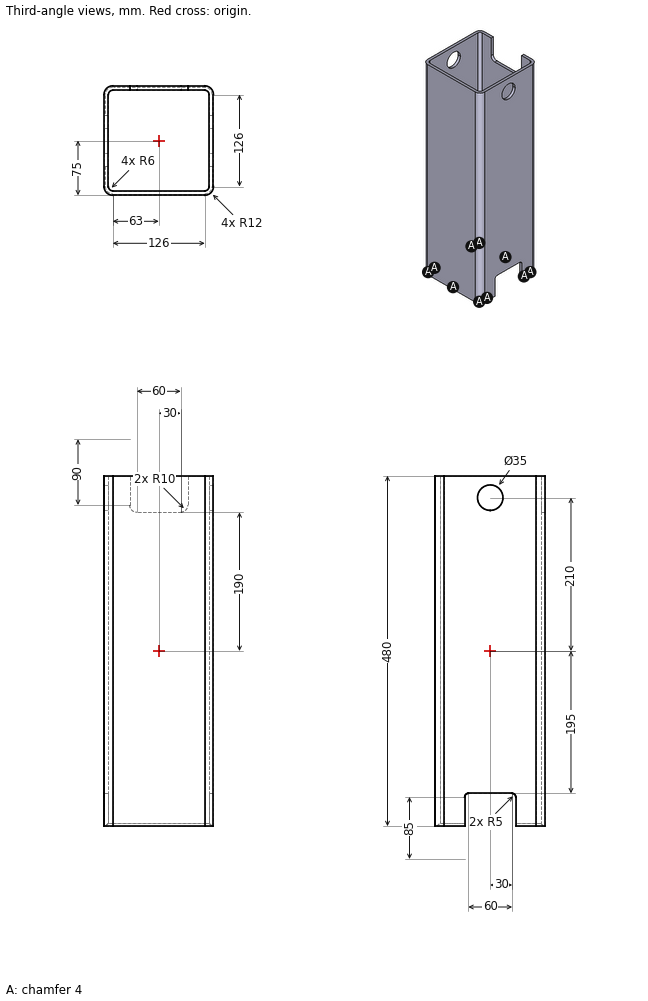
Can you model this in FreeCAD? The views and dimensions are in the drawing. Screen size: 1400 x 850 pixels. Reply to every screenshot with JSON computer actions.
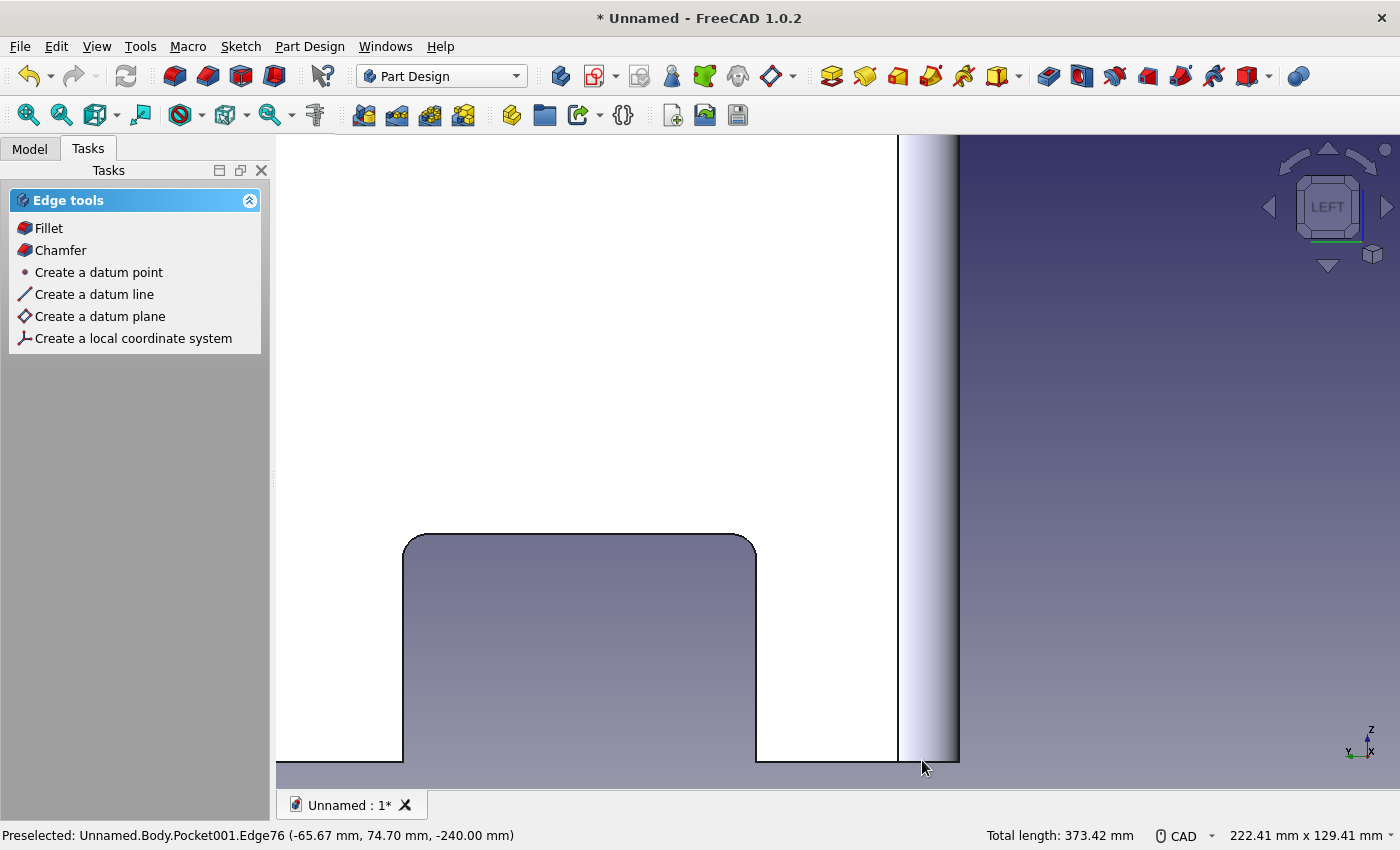
{"action": "key", "text": "v f"}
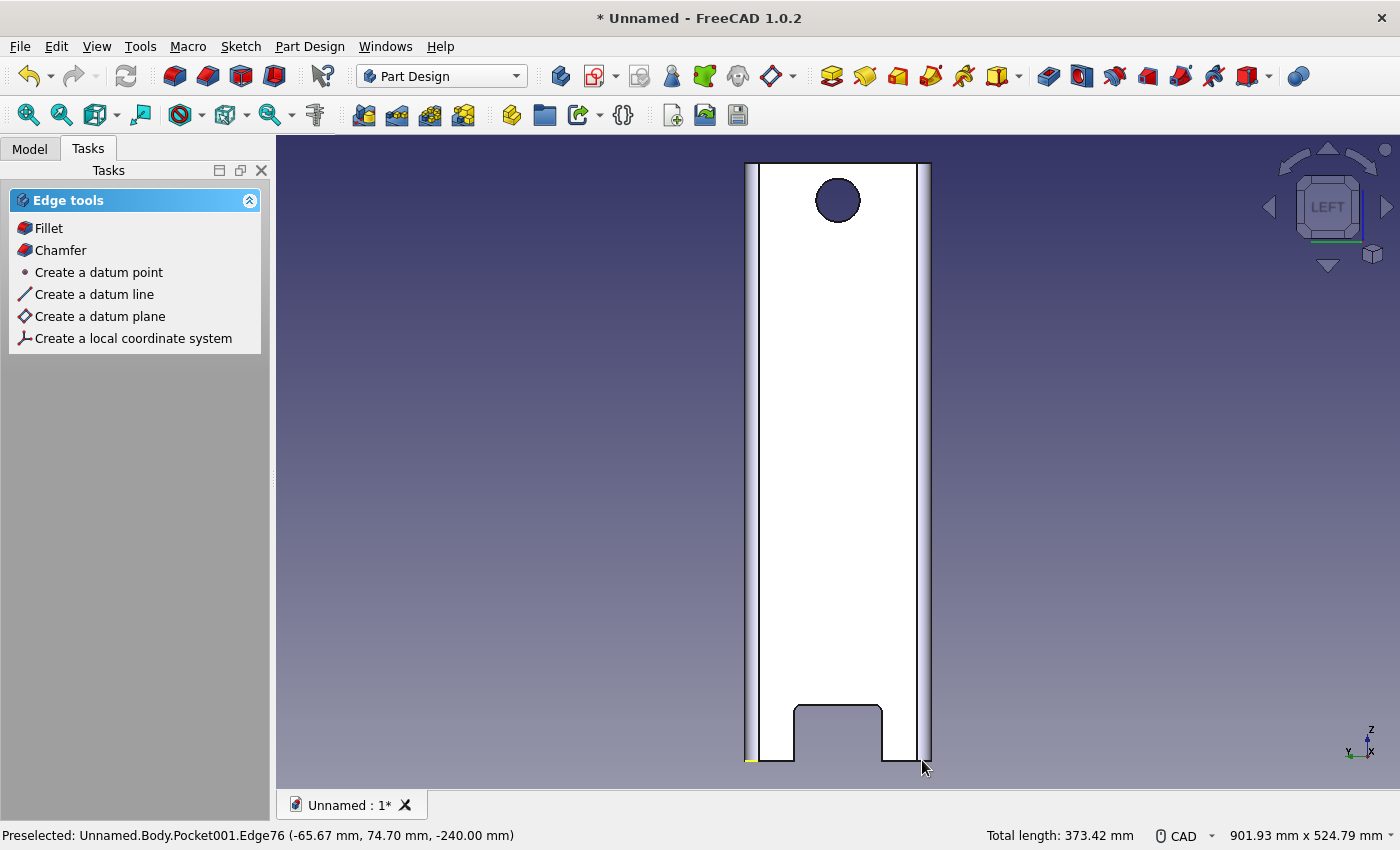
{"action": "key", "text": "v 3"}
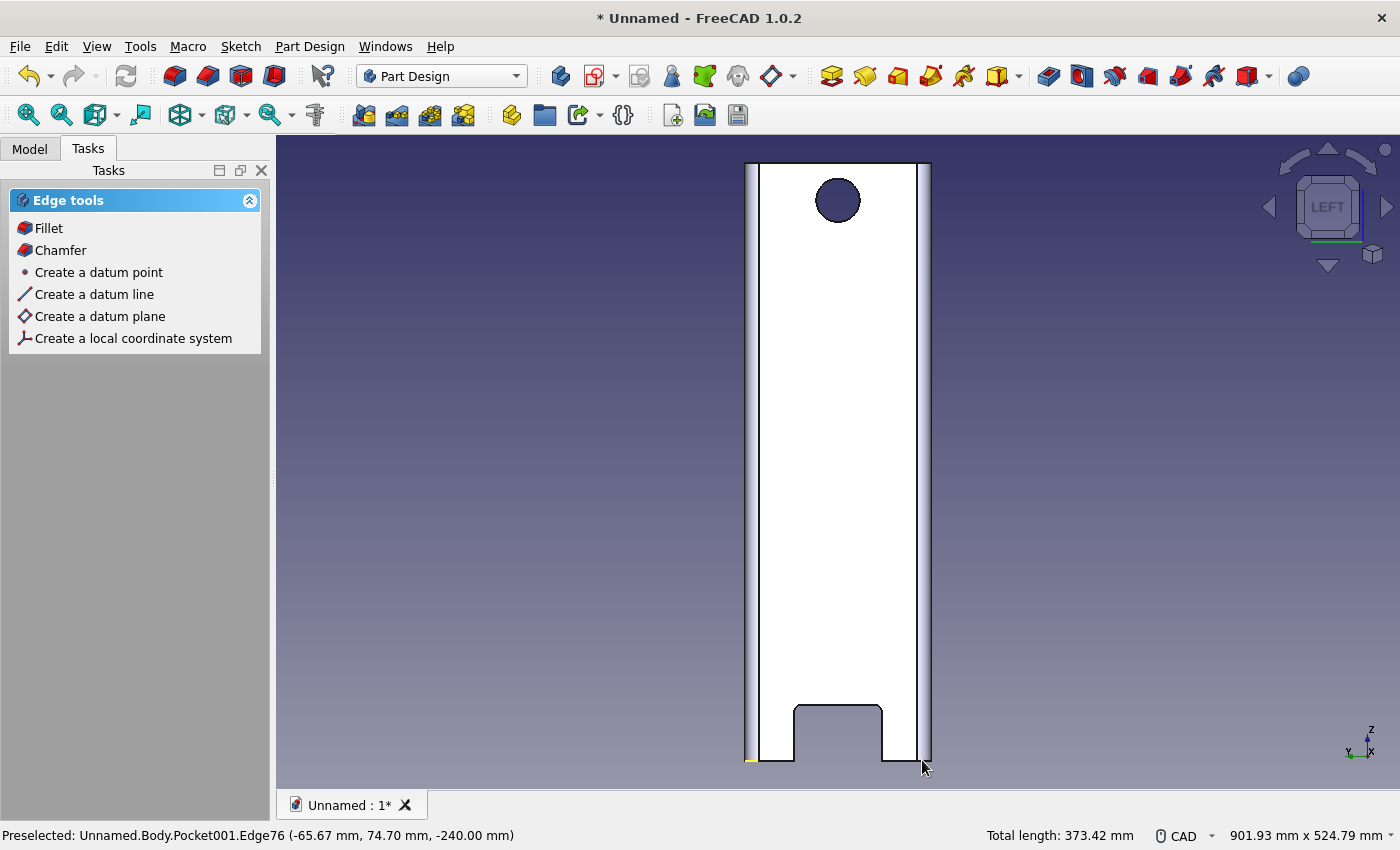
{"action": "key", "text": "0"}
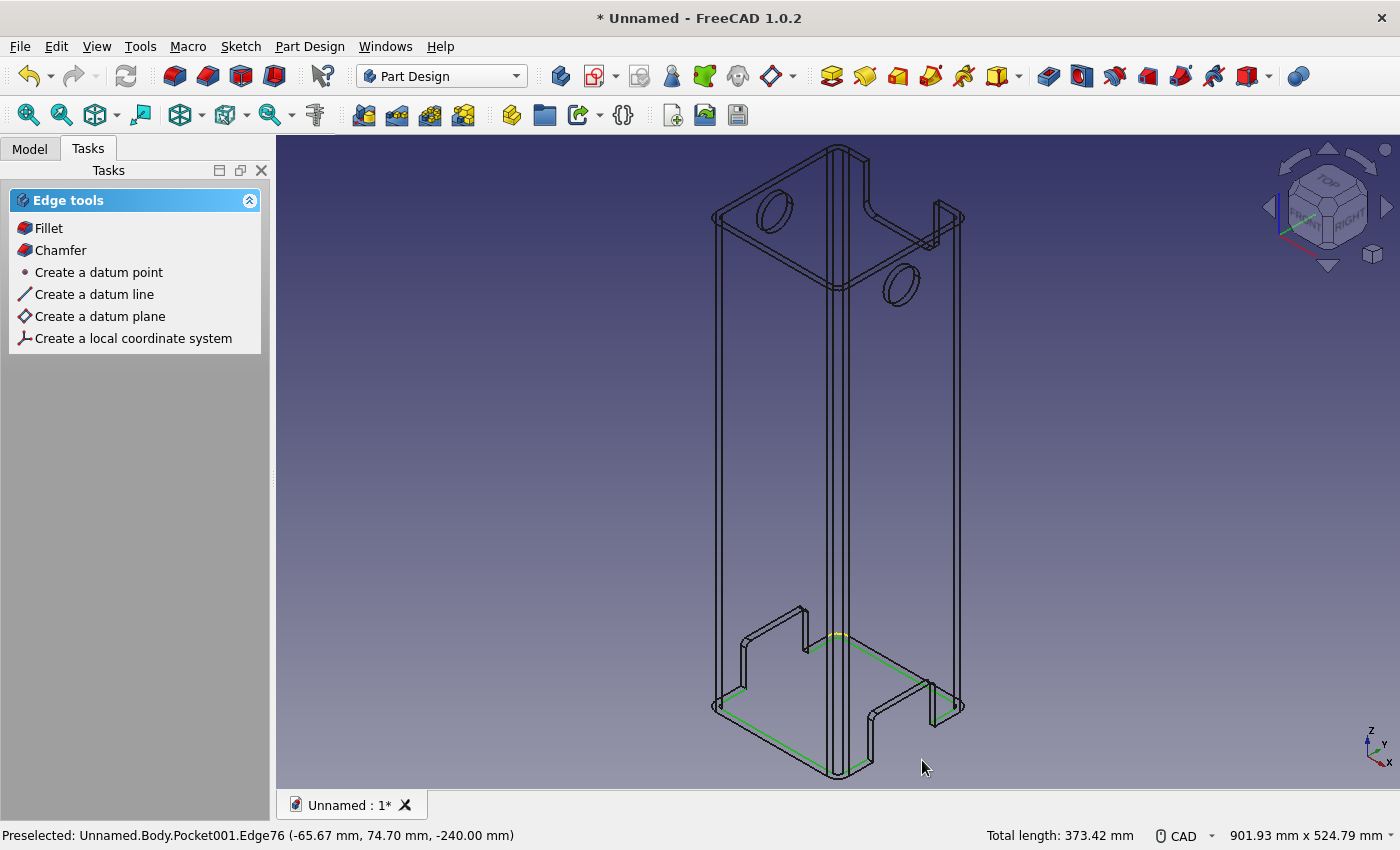
{"action": "scroll", "coordinate": [719, 705], "scroll_direction": "up", "scroll_amount": 7}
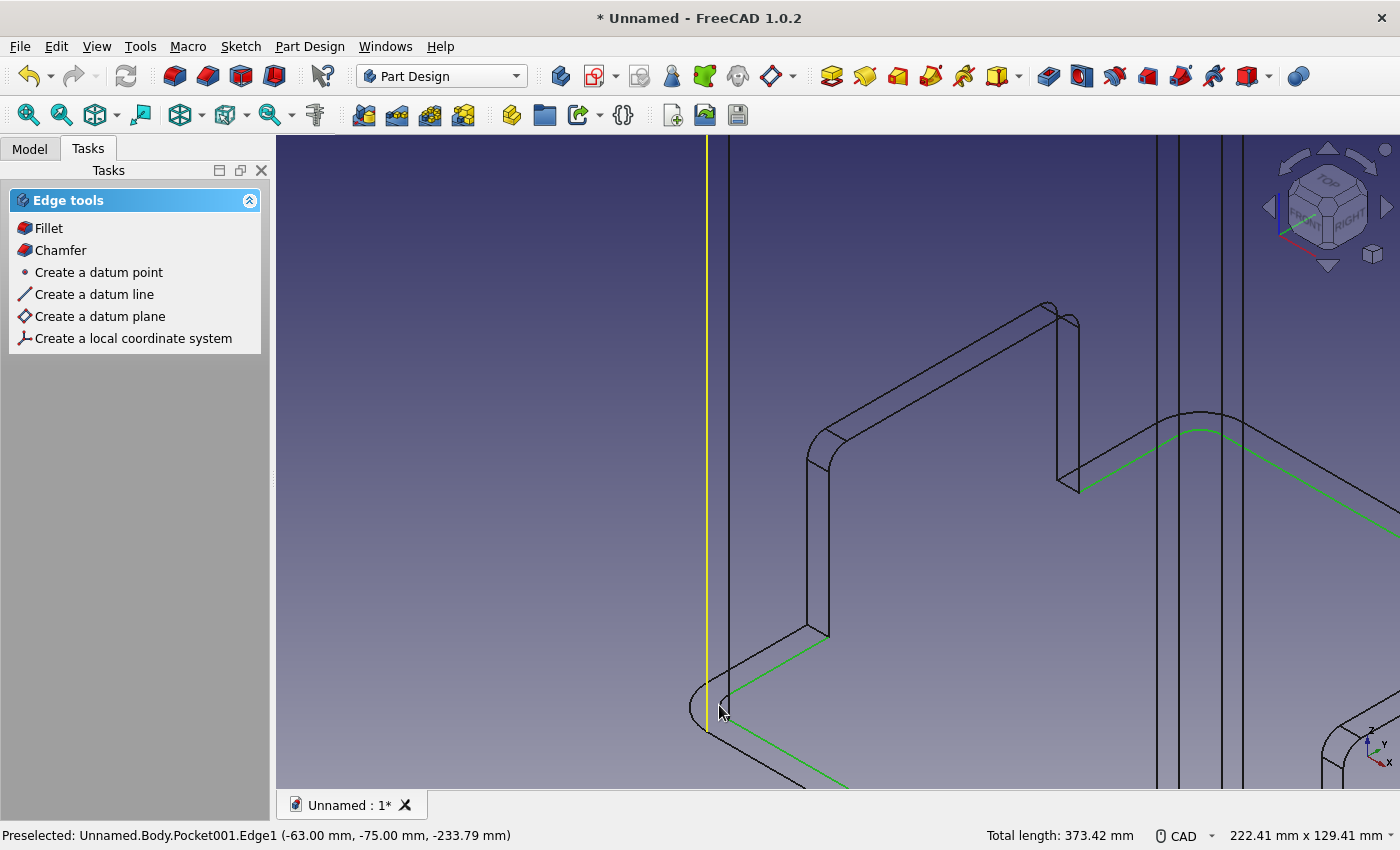
{"action": "left_click", "coordinate": [720, 706], "text": "ctrl"}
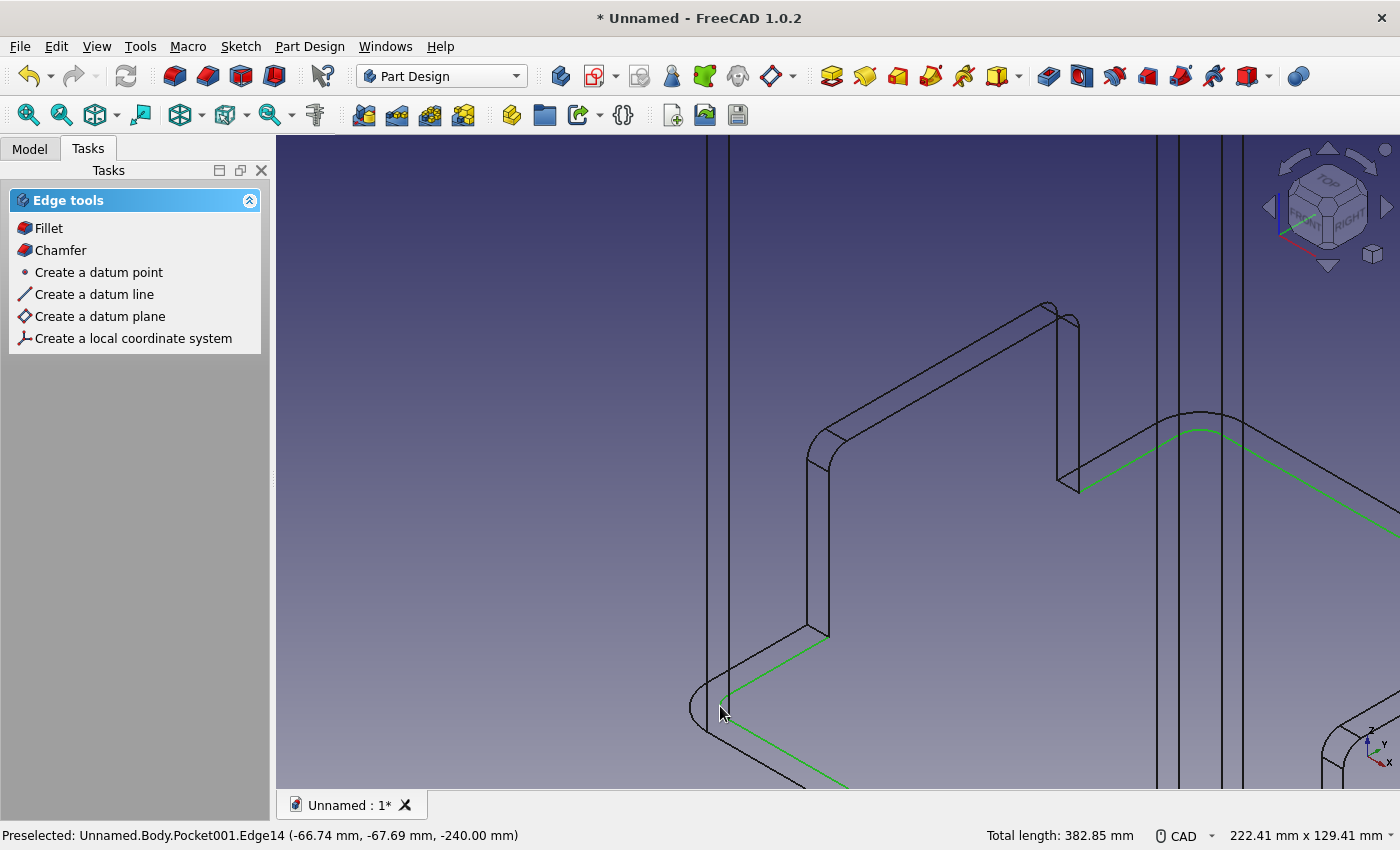
{"action": "left_click", "coordinate": [29, 116]}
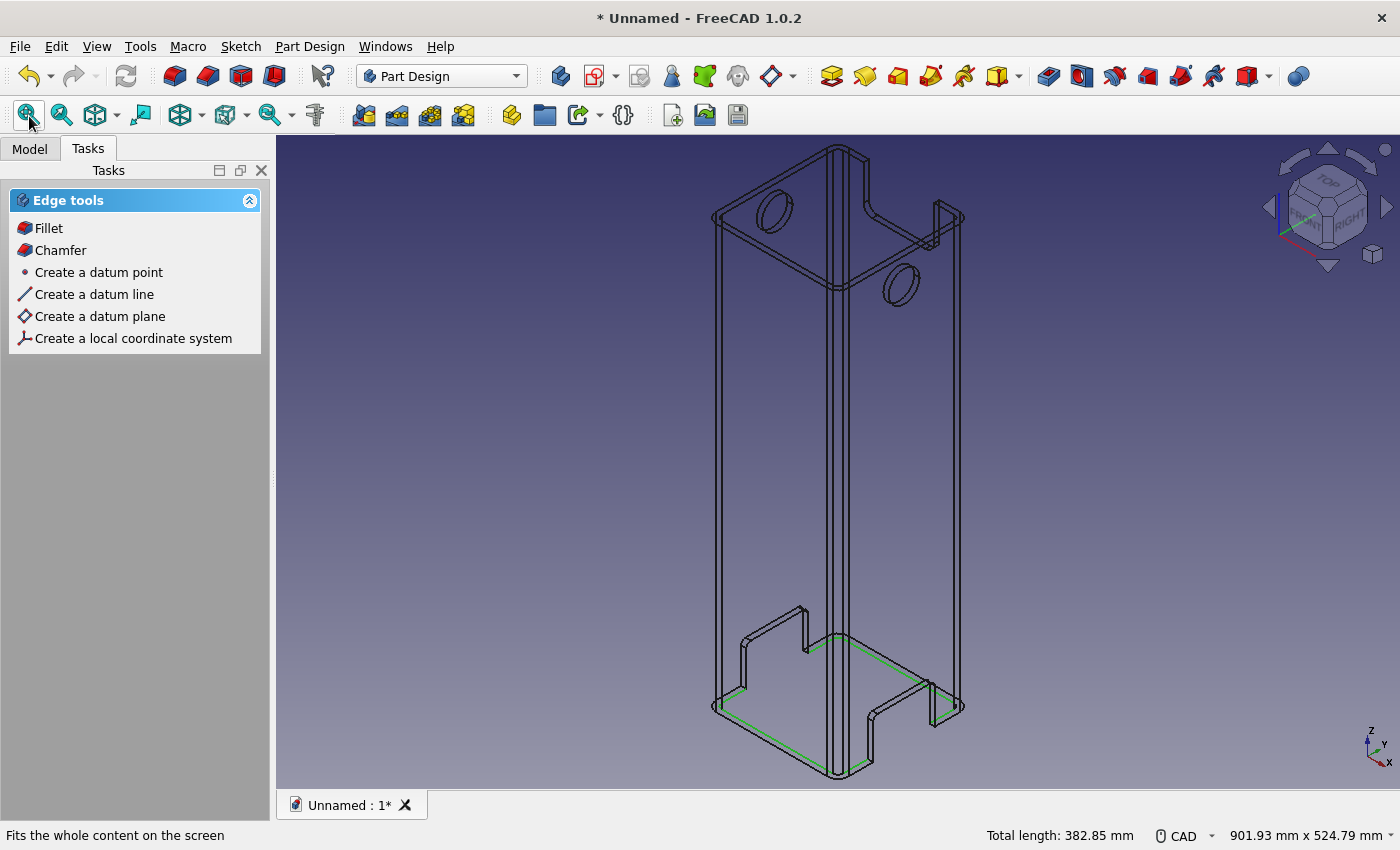
{"action": "key", "text": "2"}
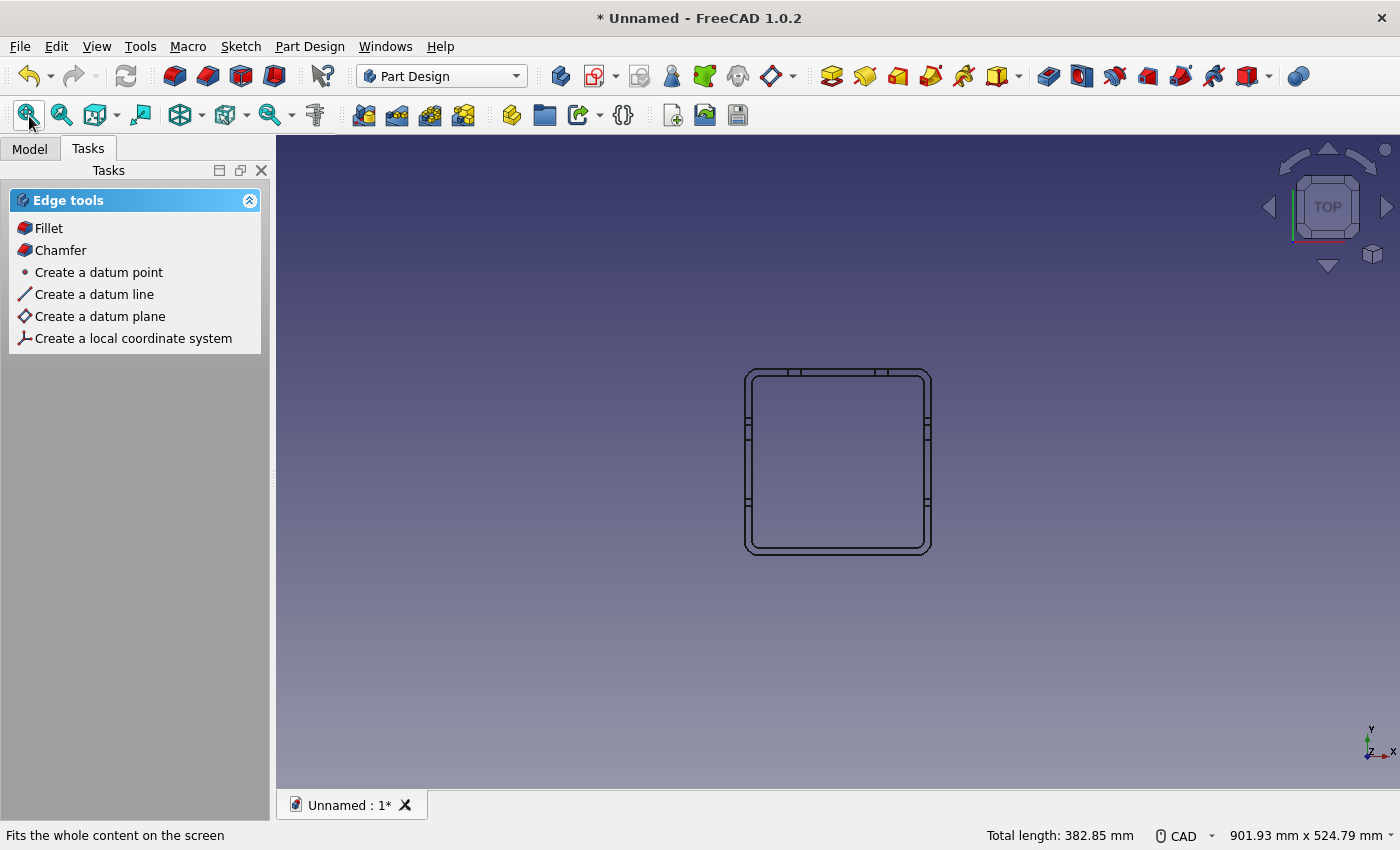
{"action": "key", "text": "v f"}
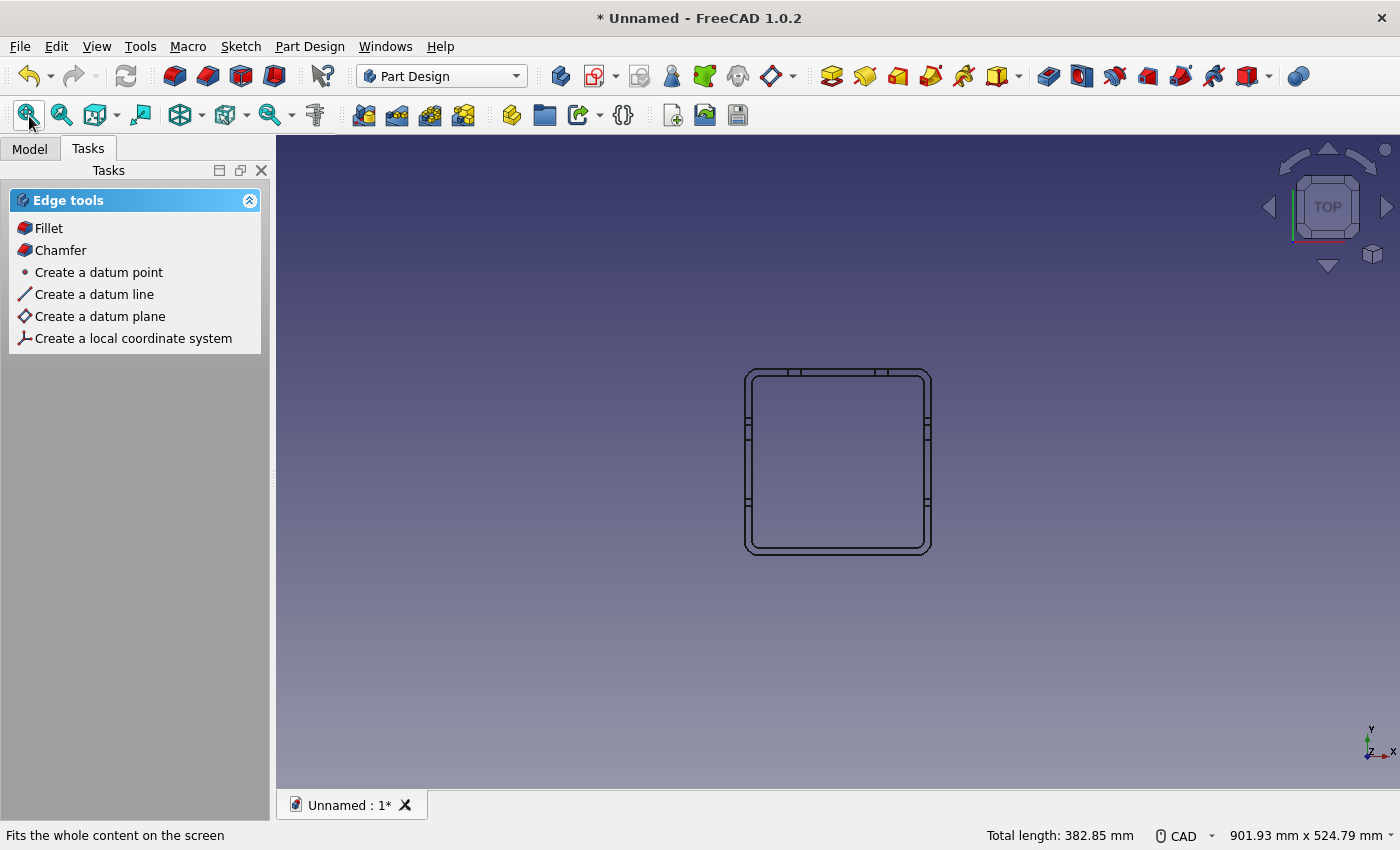
{"action": "scroll", "coordinate": [922, 545], "scroll_direction": "up", "scroll_amount": 7}